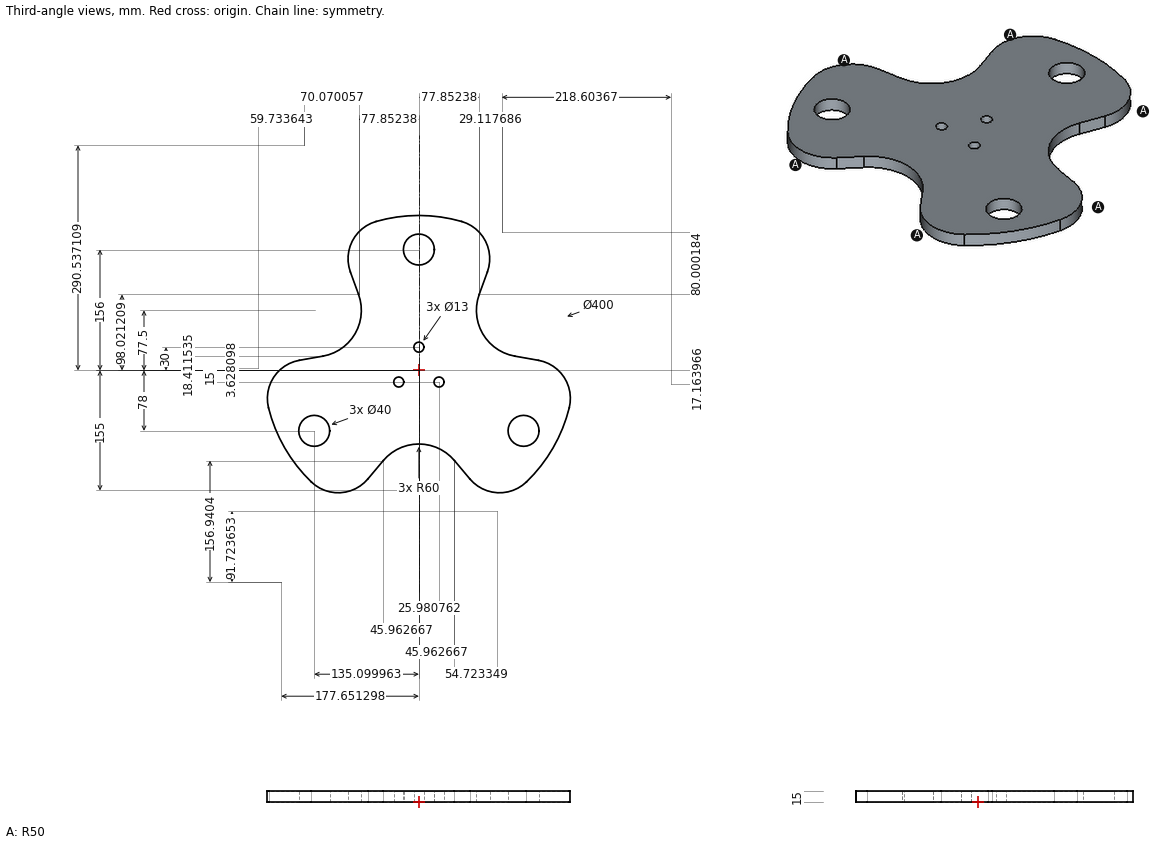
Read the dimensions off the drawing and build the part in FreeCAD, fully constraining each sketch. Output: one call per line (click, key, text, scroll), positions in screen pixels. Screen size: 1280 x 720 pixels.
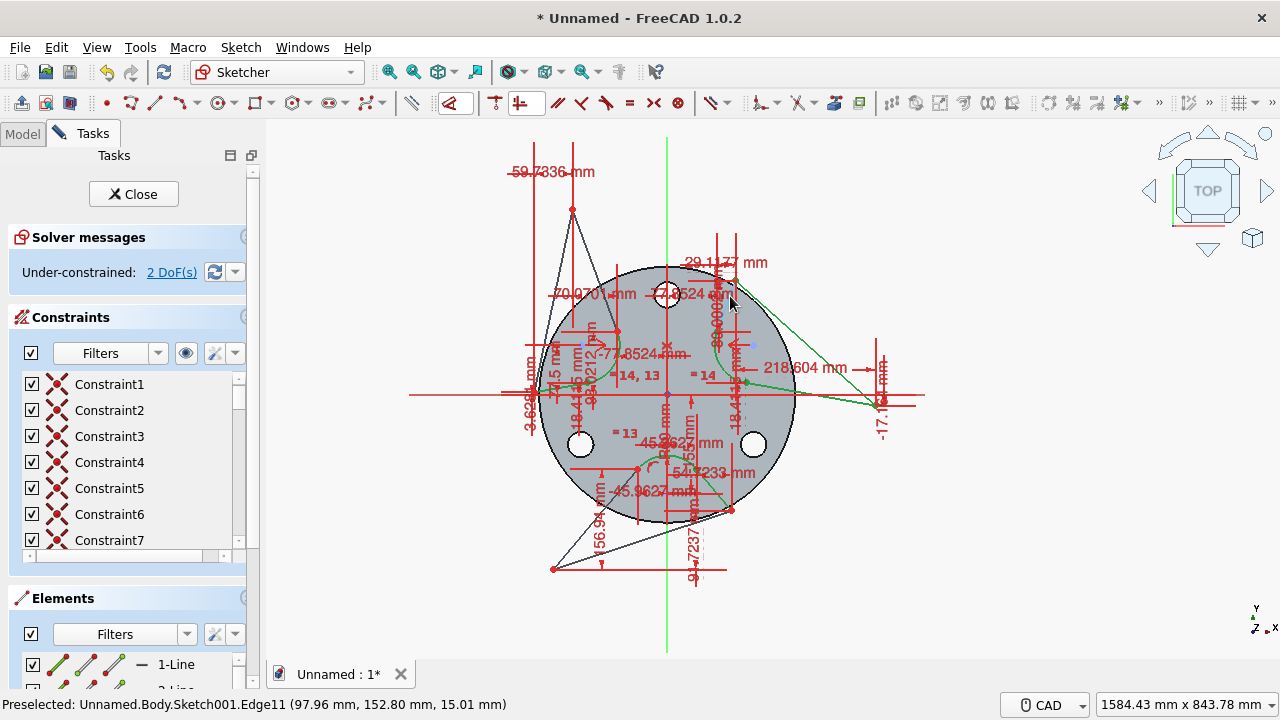
click(553, 570)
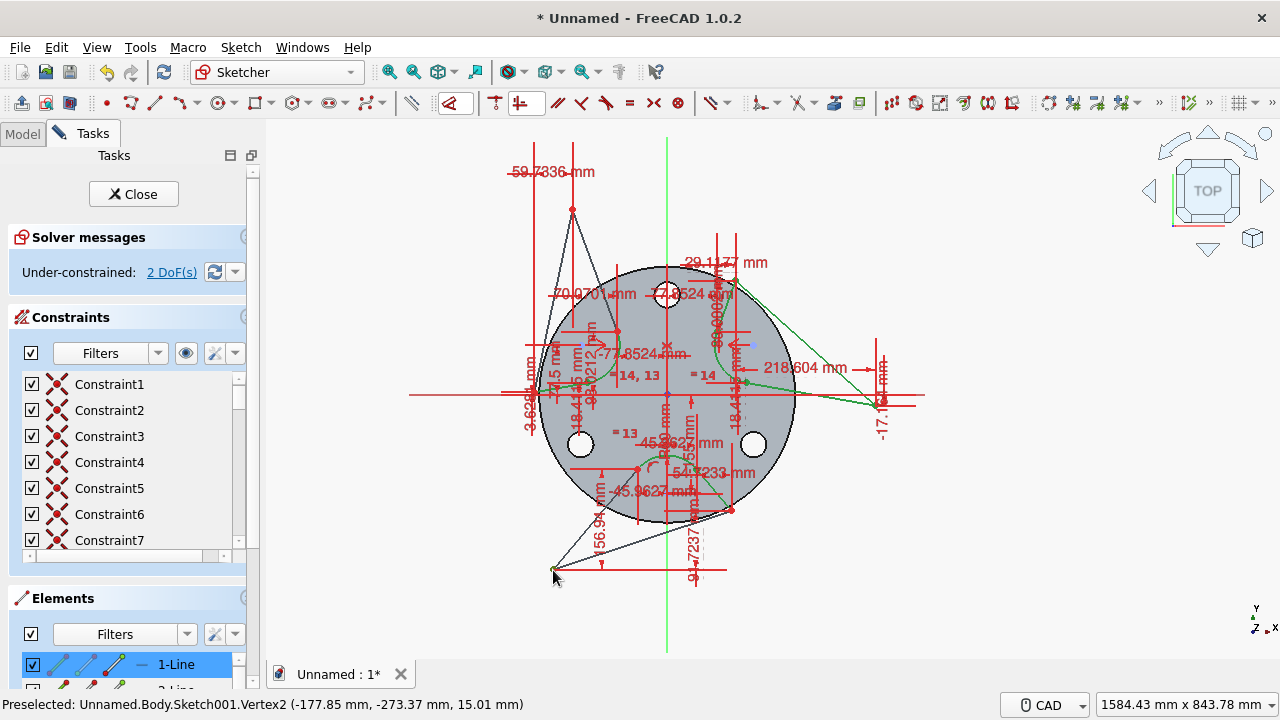
click(468, 104)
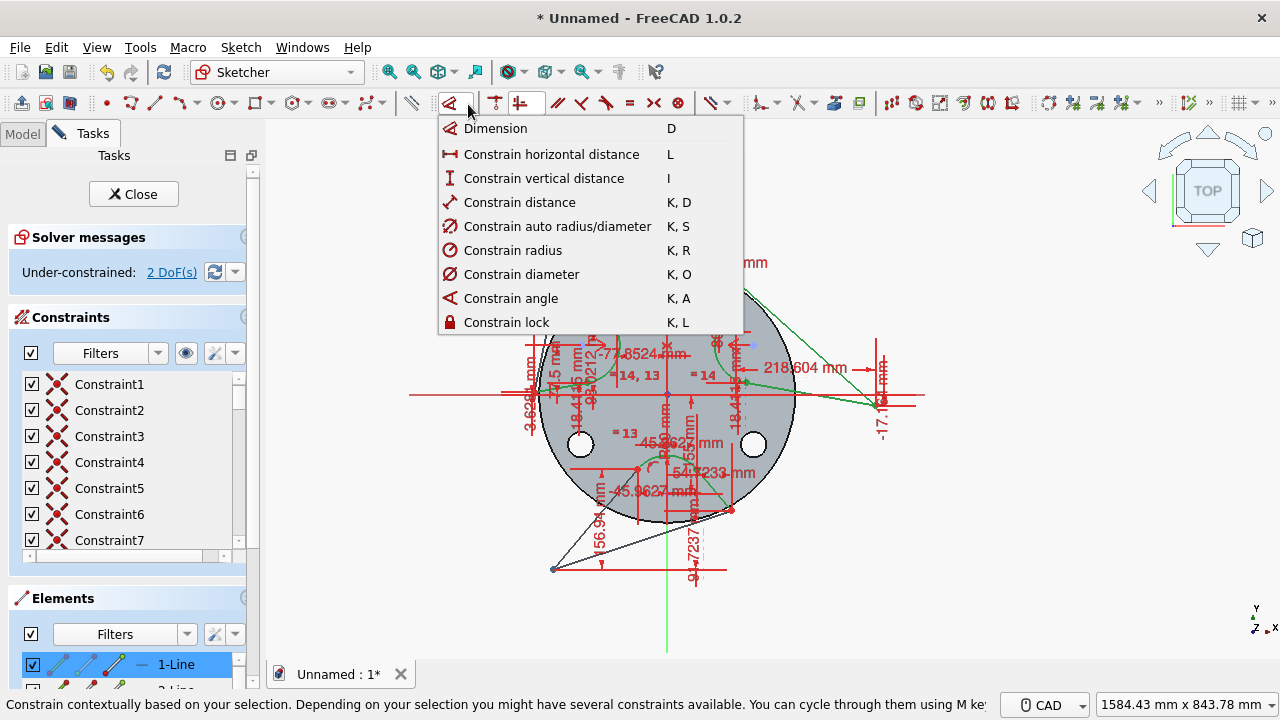
click(591, 154)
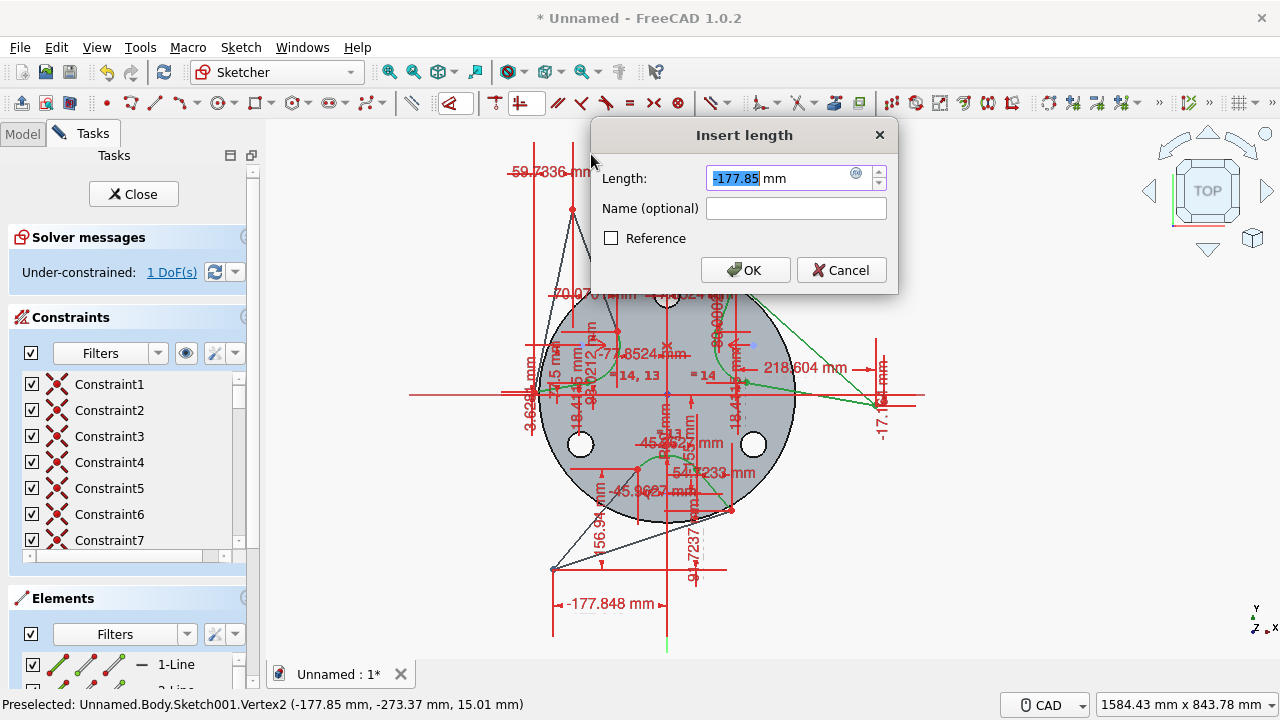
text(-177.651298)
key(Return)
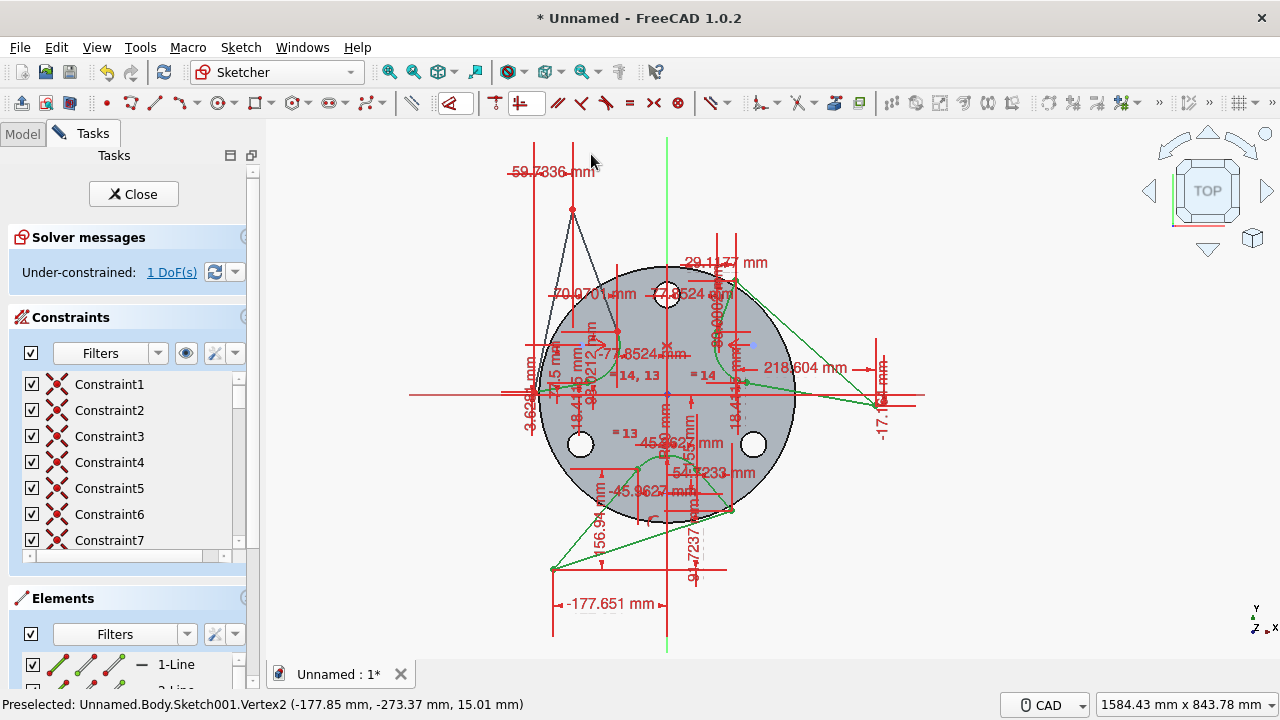
click(573, 210)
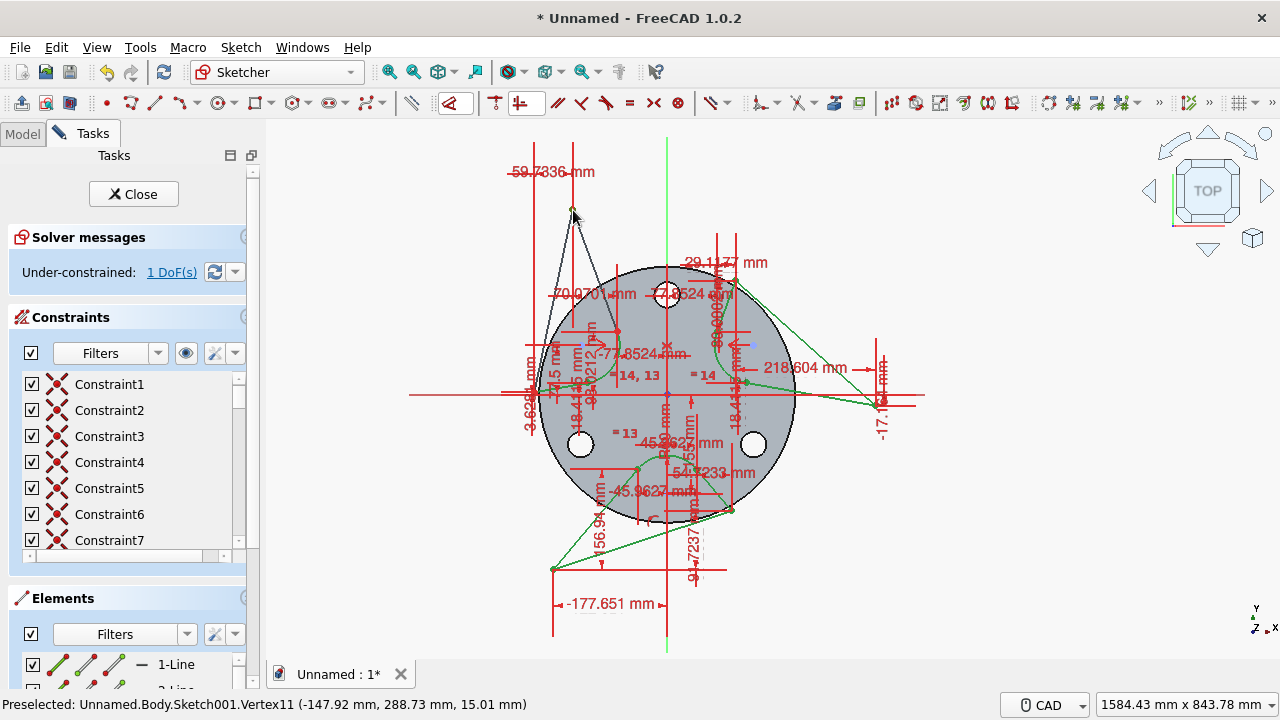
key(i)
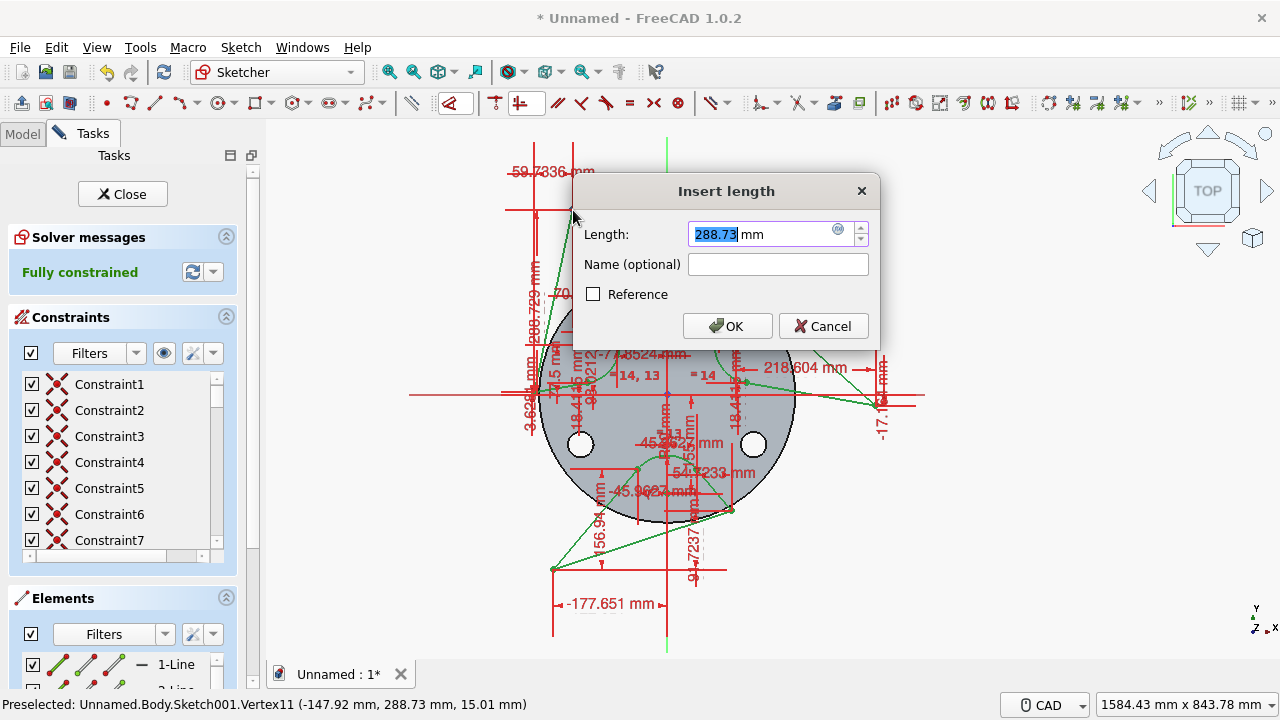
text(290.537109)
key(Return)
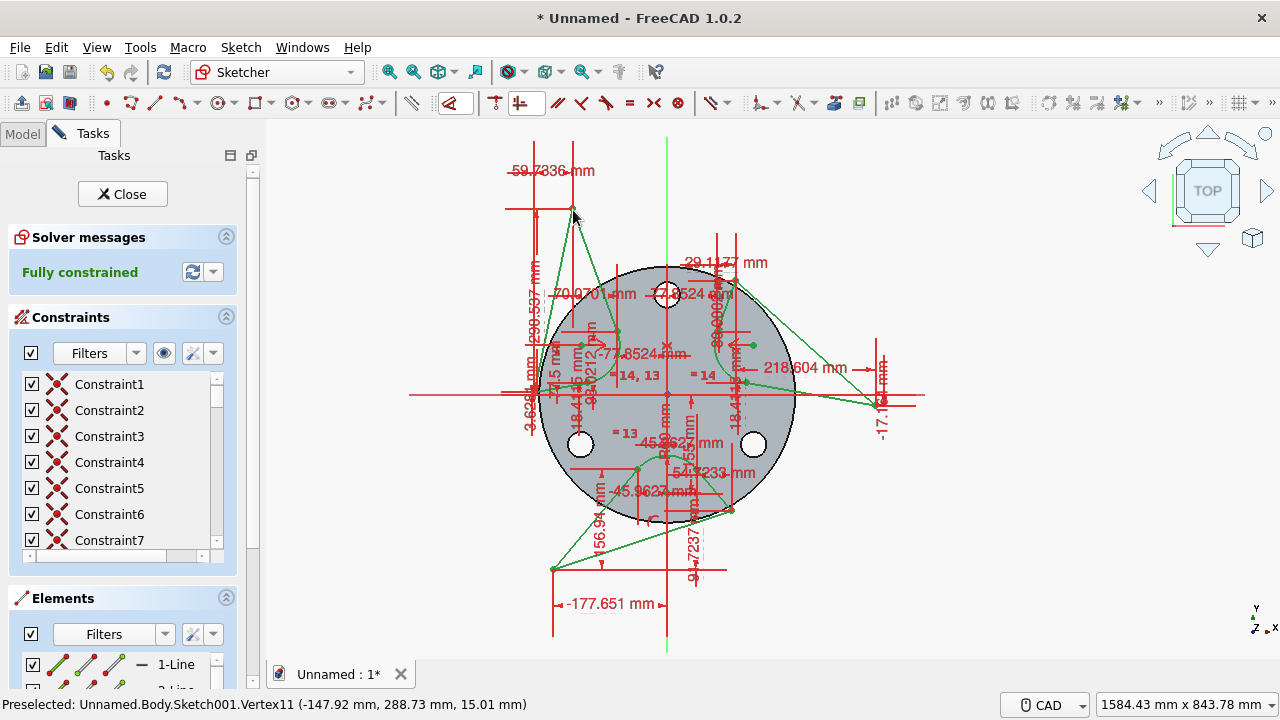
click(123, 194)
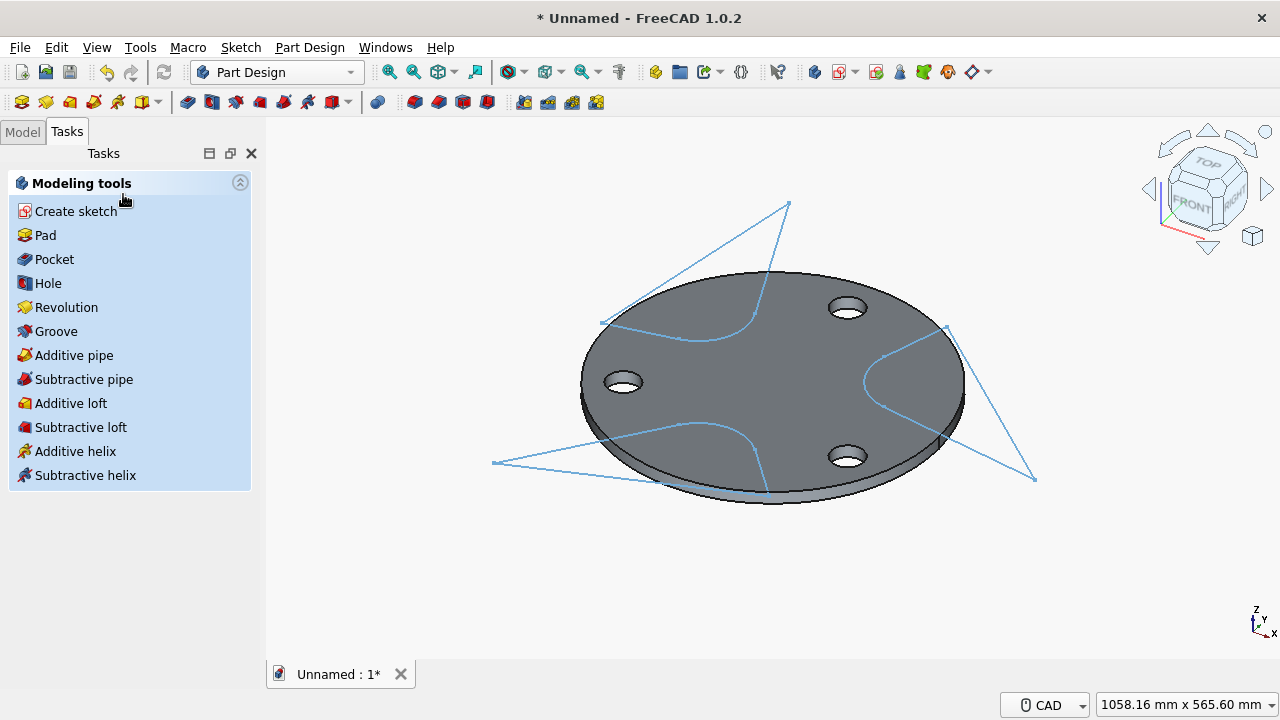
click(188, 102)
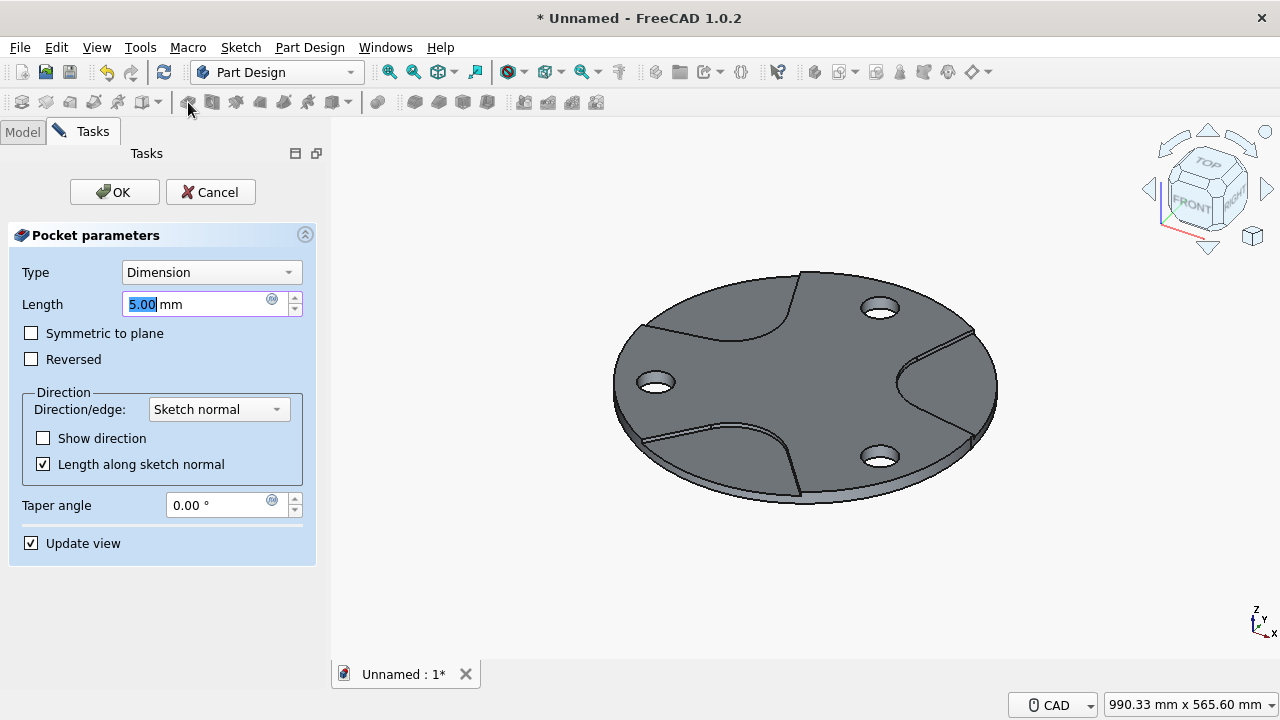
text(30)
key(Tab)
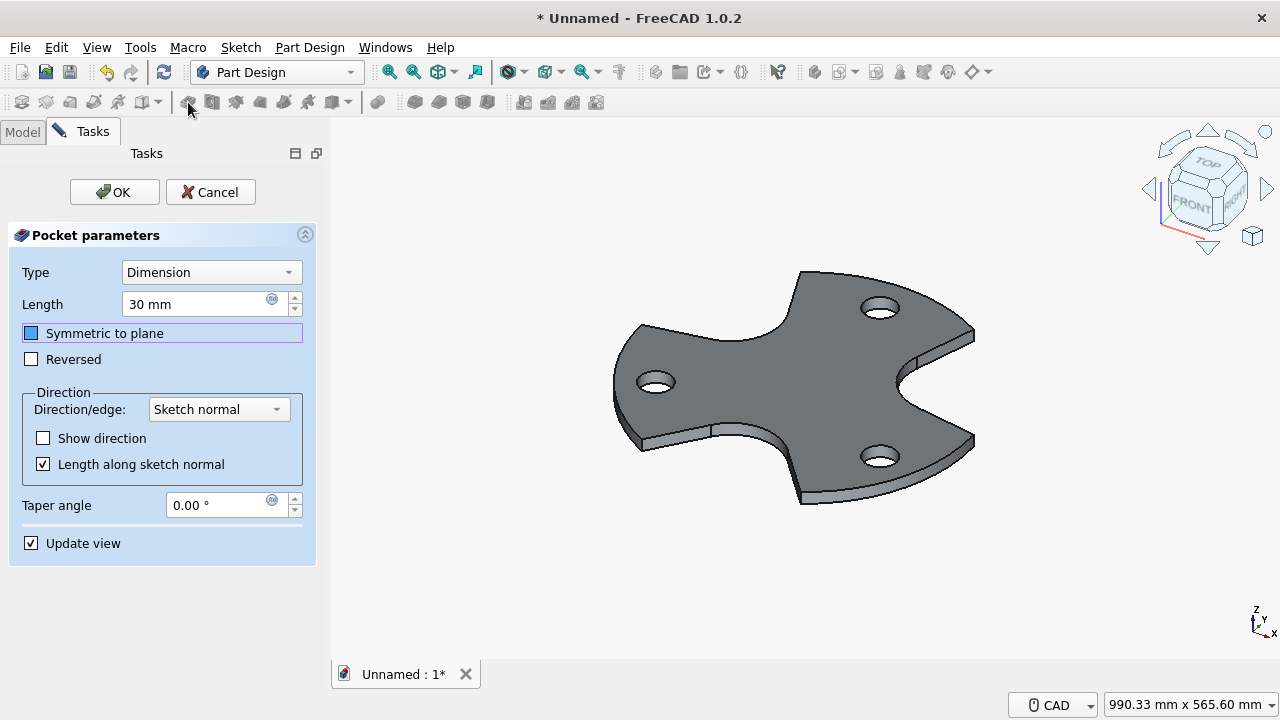
click(115, 192)